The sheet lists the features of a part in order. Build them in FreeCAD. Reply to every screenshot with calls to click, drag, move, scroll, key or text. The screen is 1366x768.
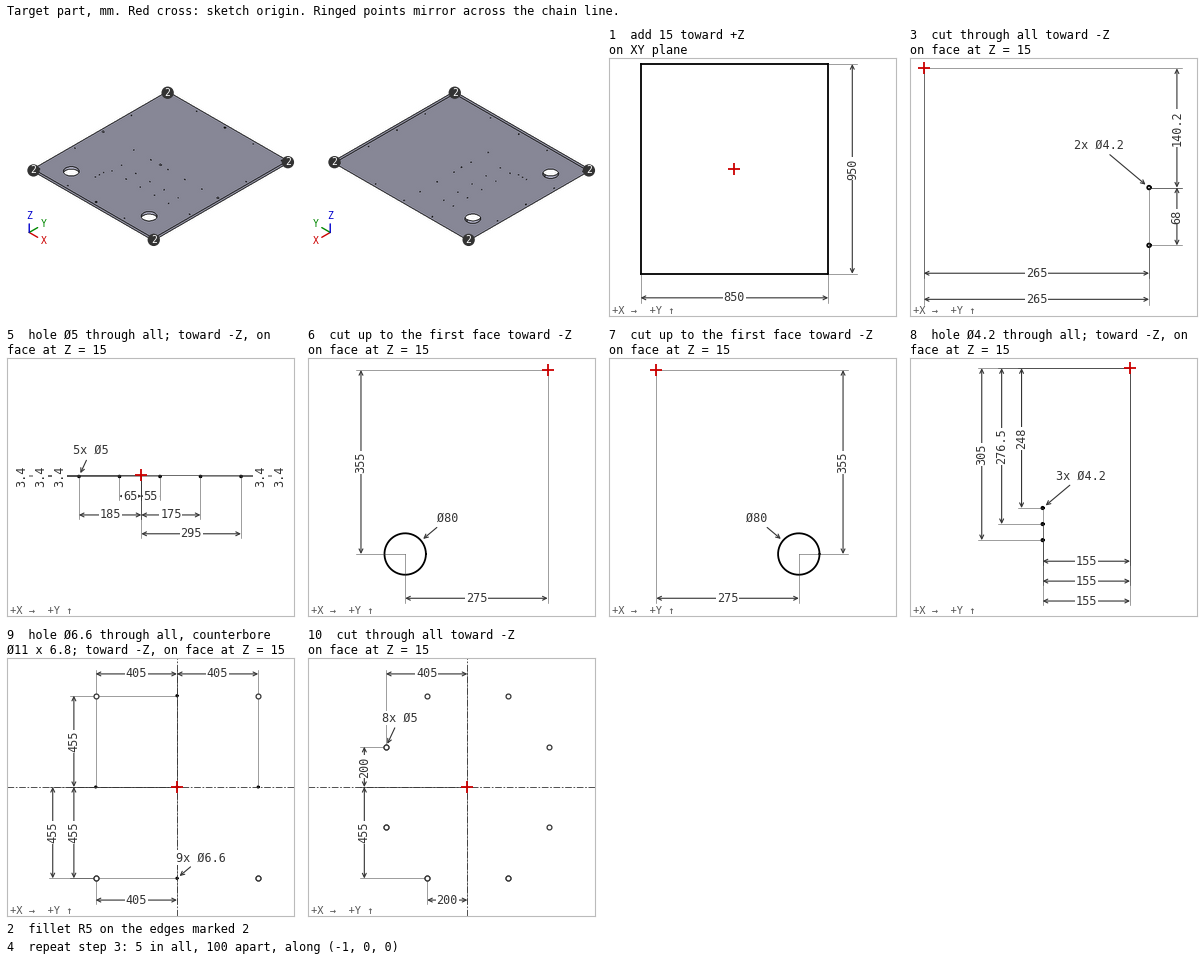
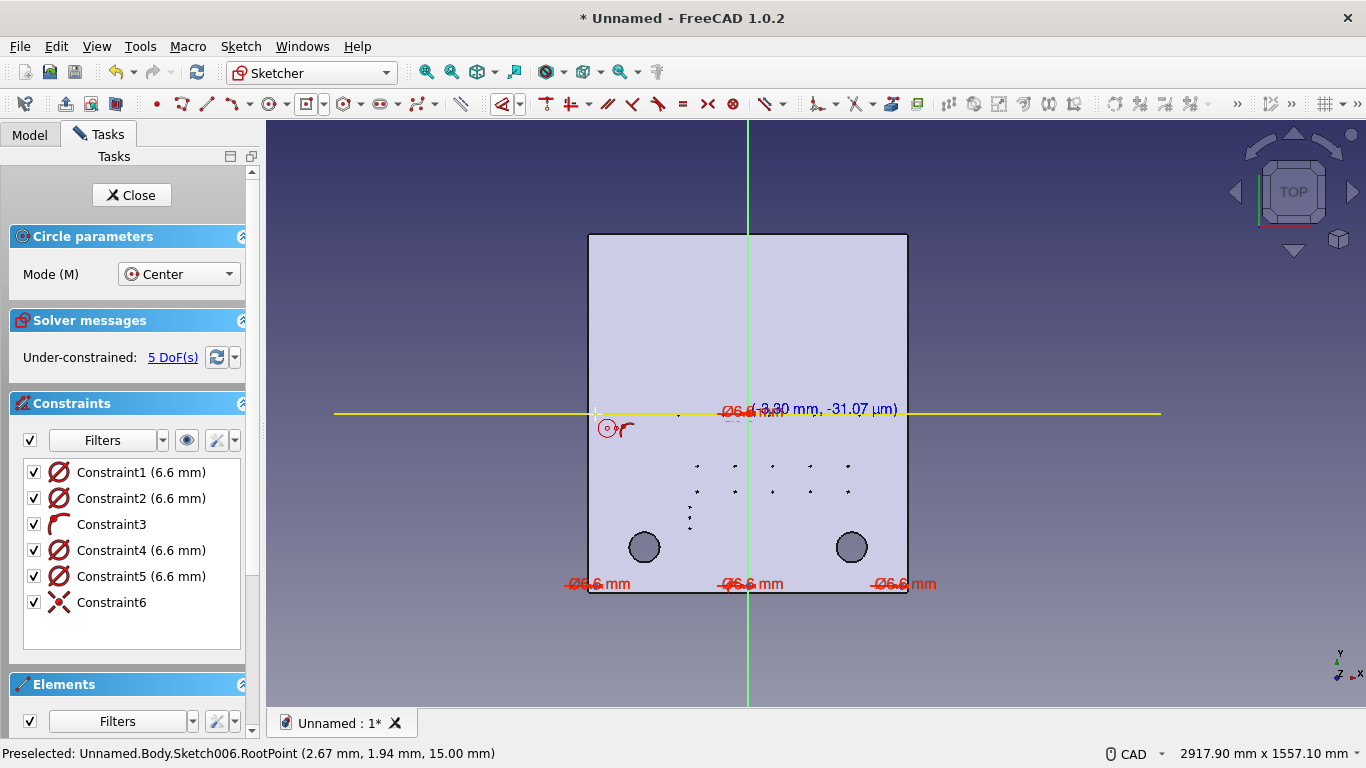
click(595, 414)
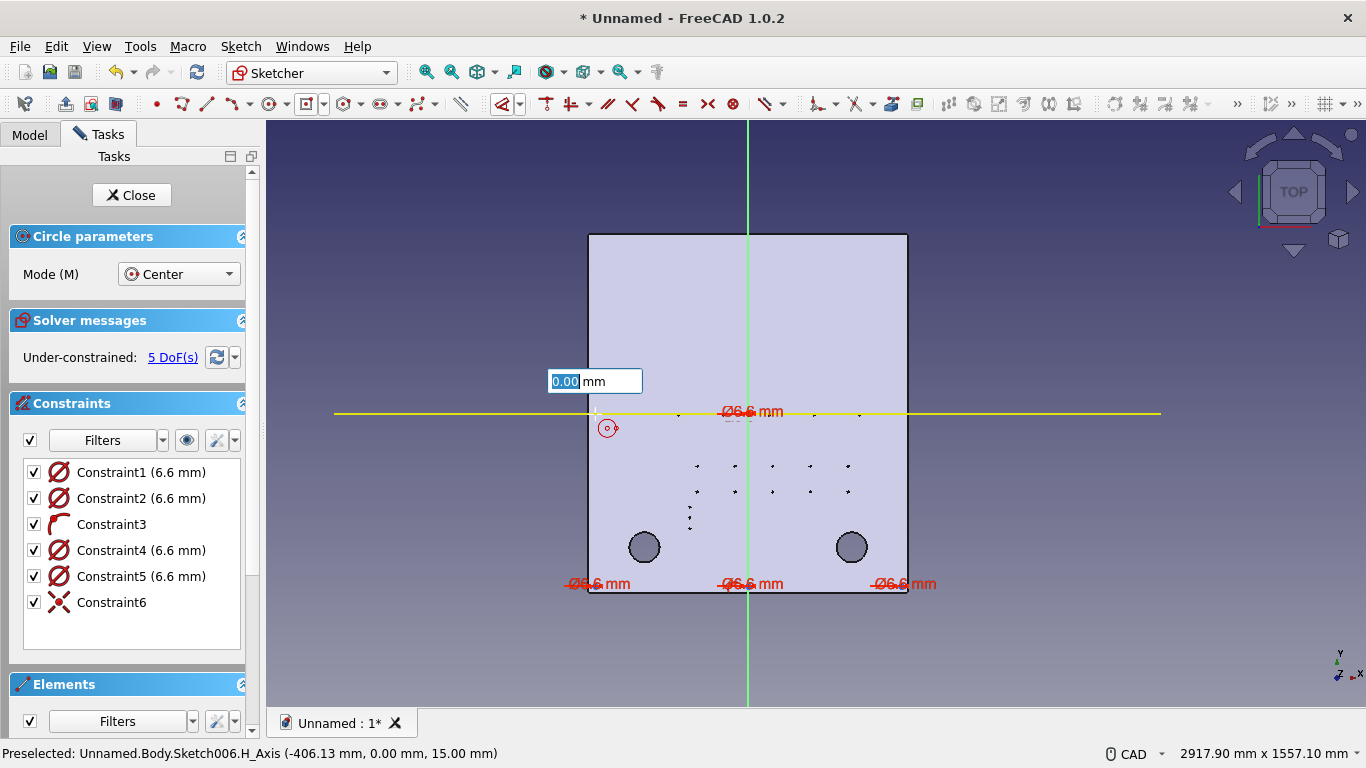
scroll(596, 412, up, 14)
move(589, 411)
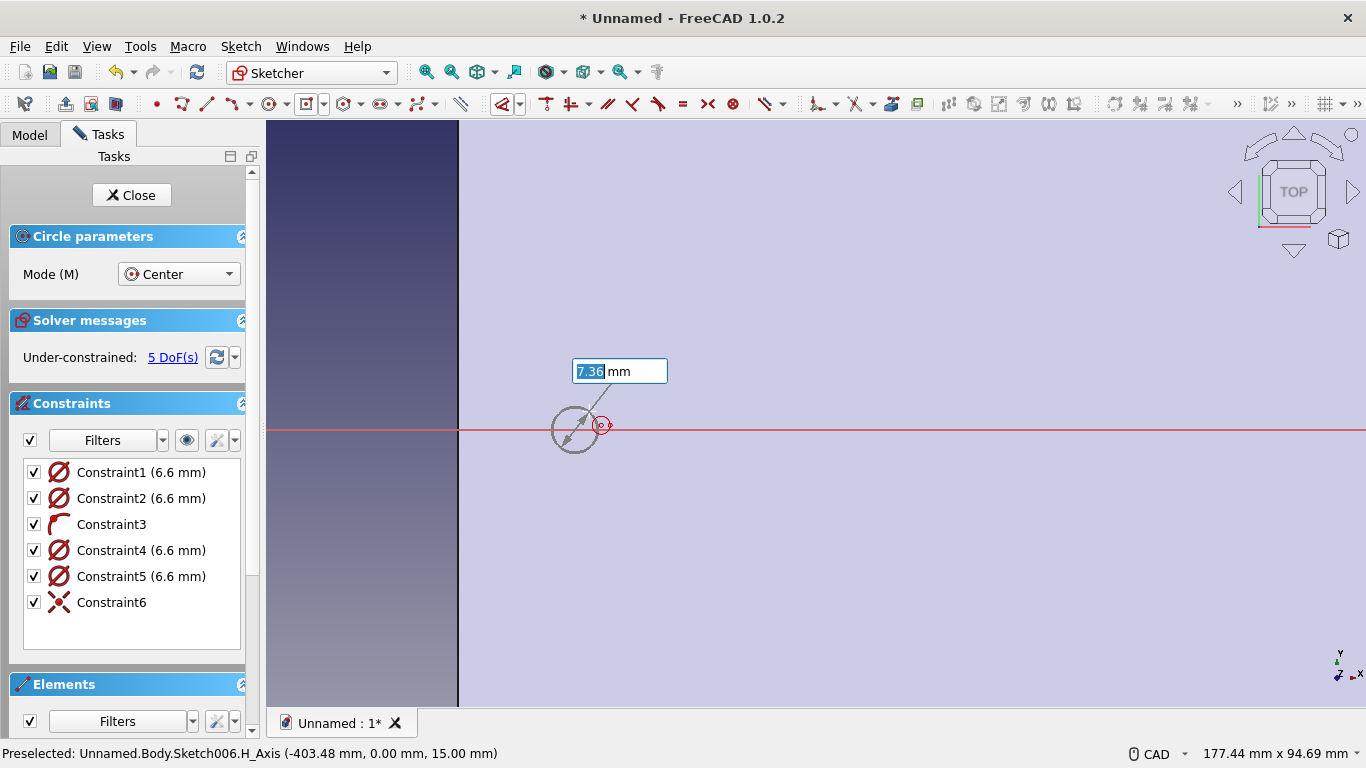
text(6.6)
key(Return)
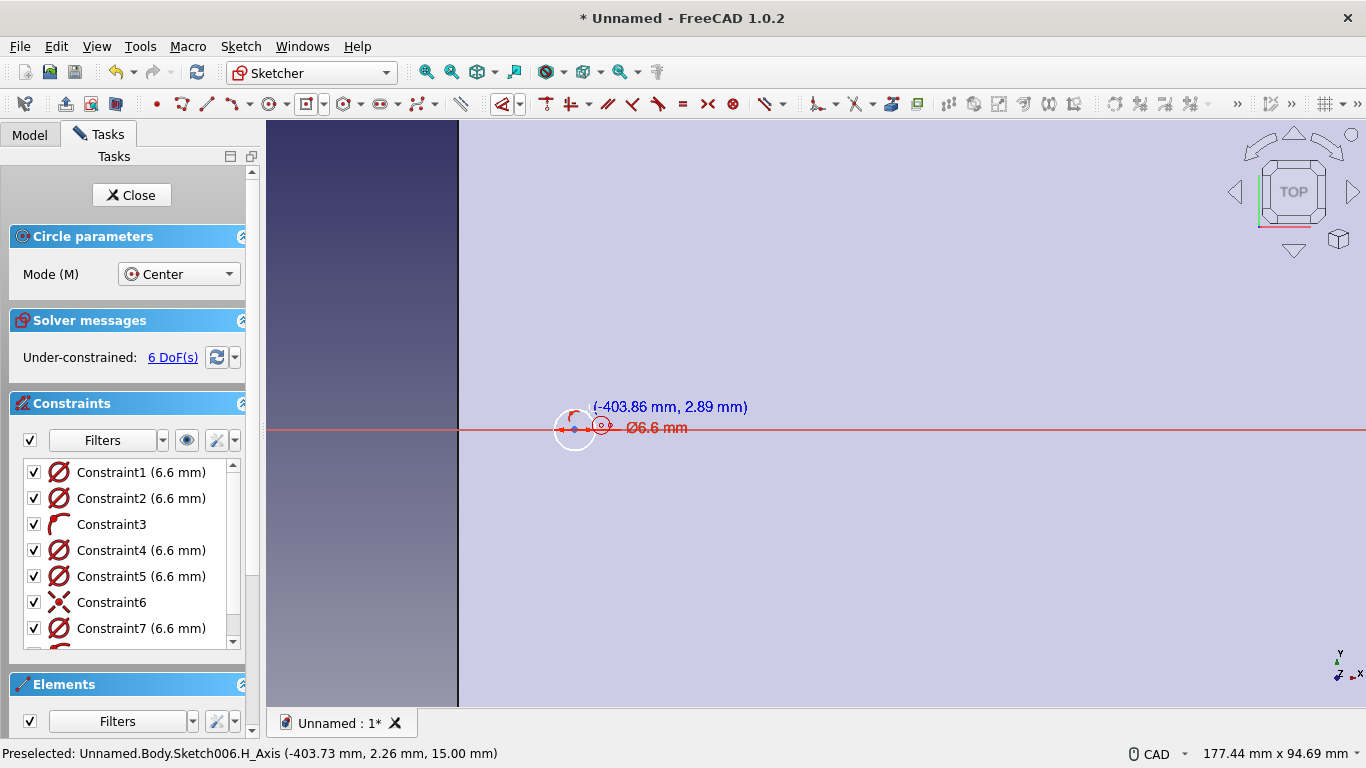
scroll(596, 412, down, 14)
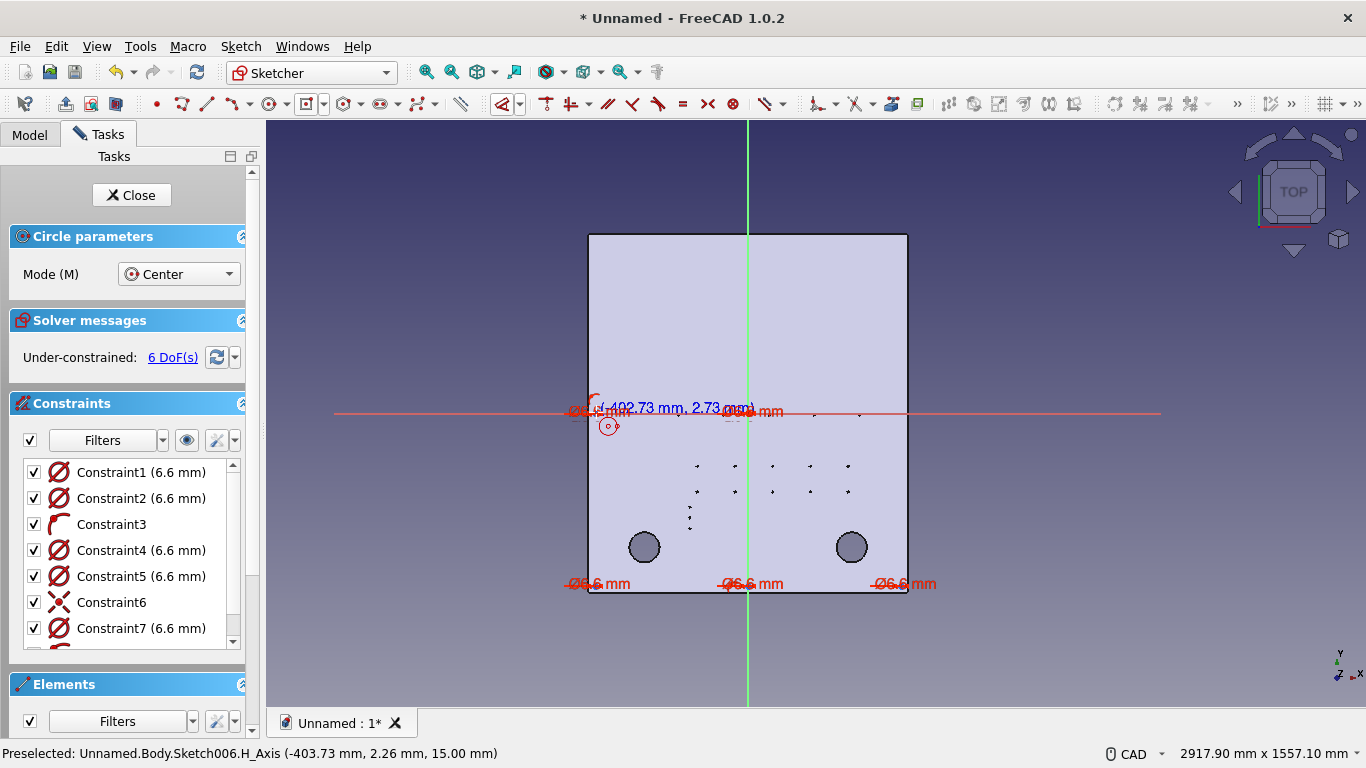
scroll(595, 242, up, 15)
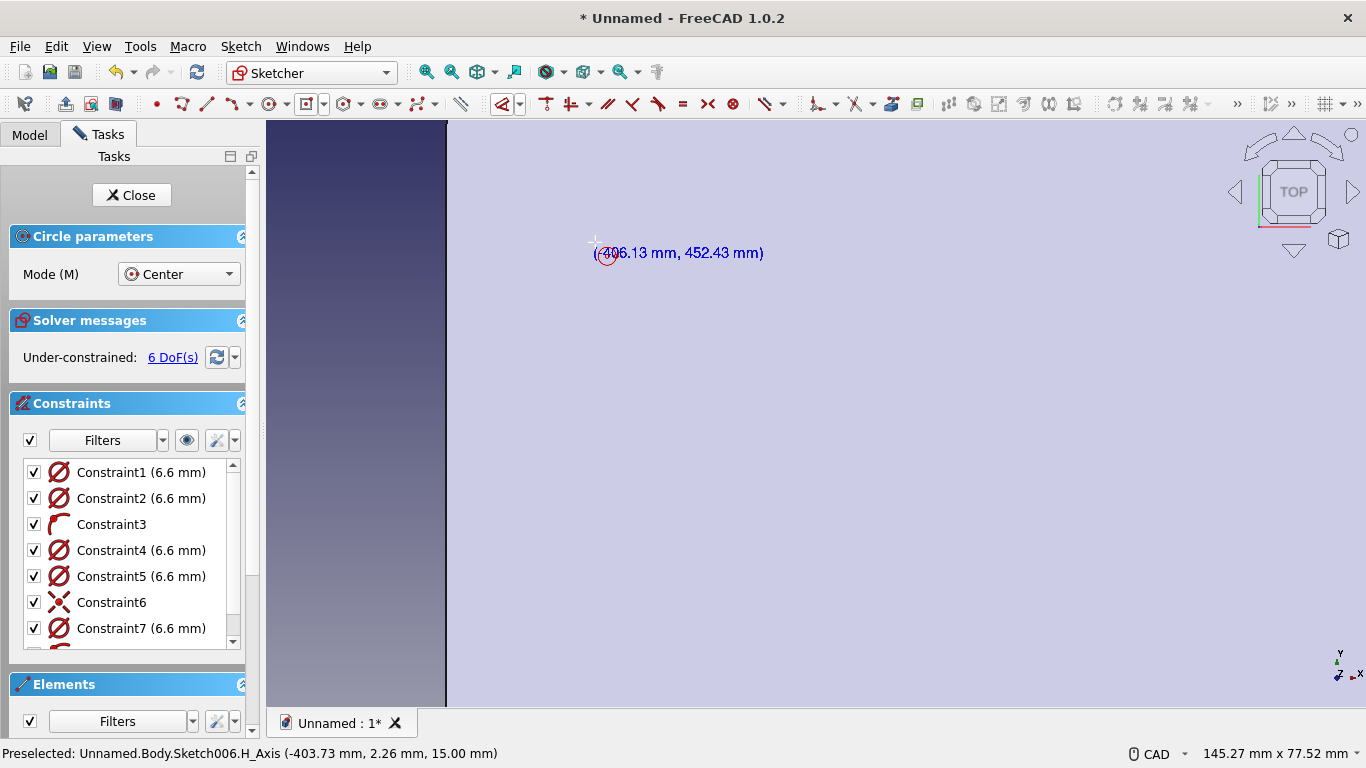
scroll(595, 242, down, 15)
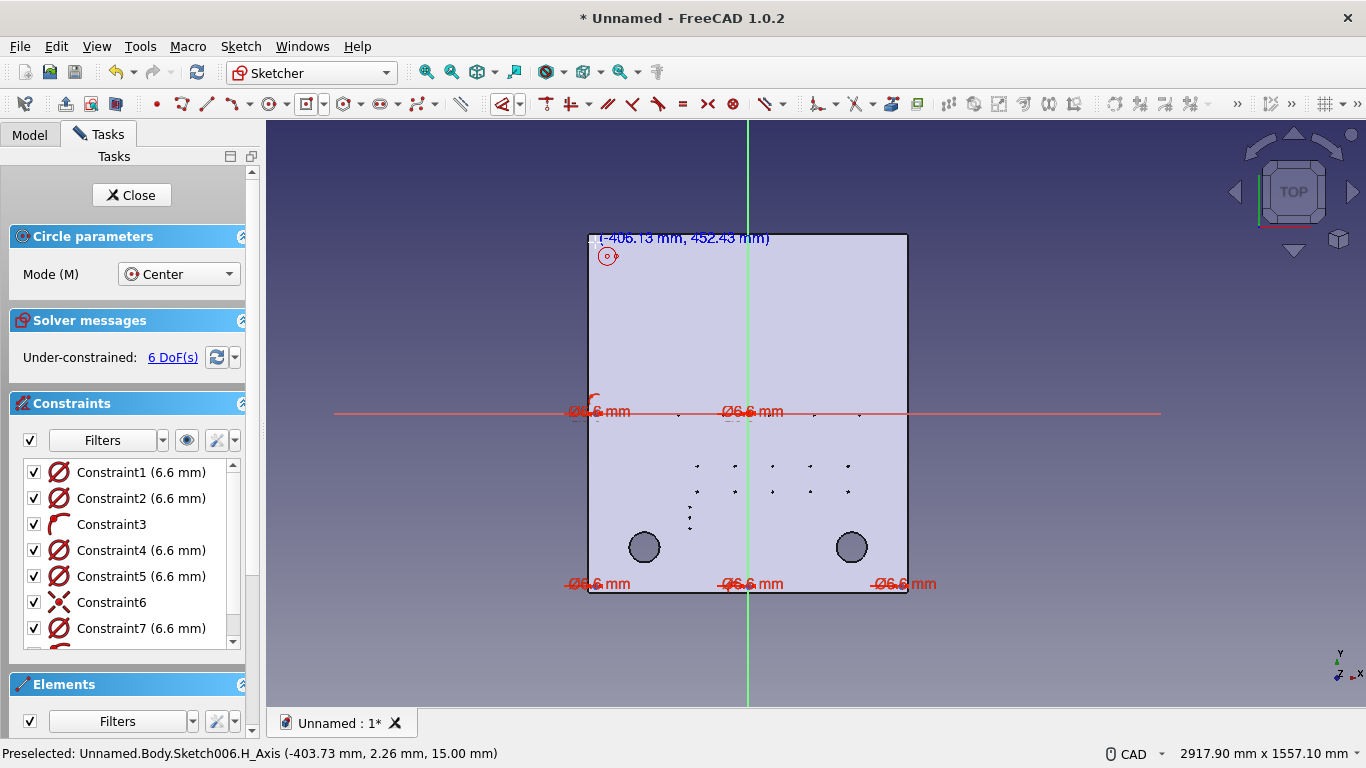
click(595, 242)
move(596, 241)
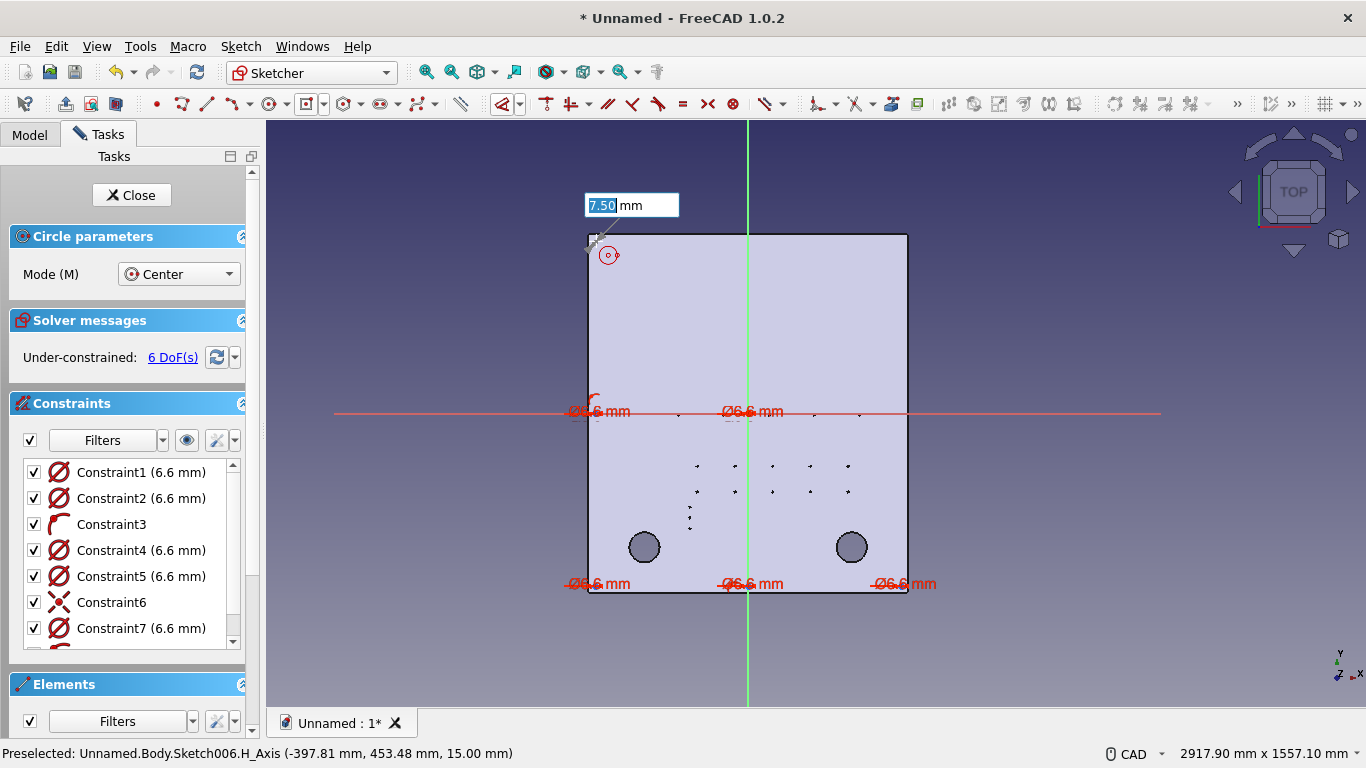
text(6.6)
key(Return)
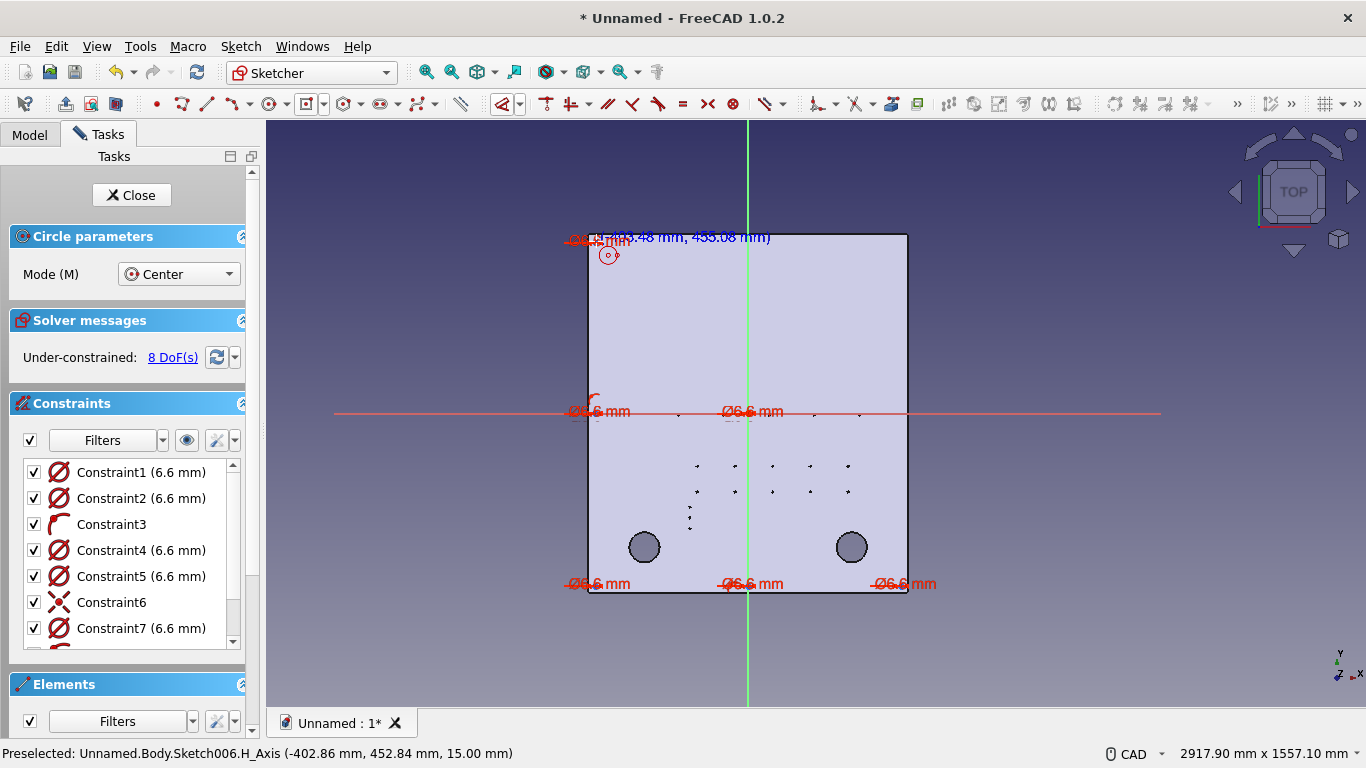
scroll(748, 242, up, 15)